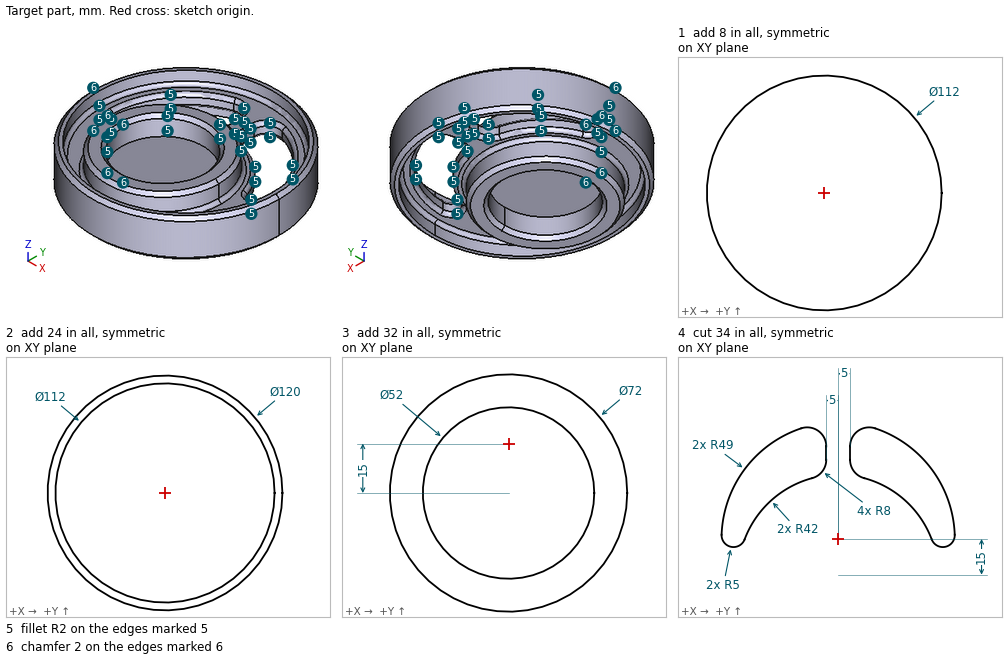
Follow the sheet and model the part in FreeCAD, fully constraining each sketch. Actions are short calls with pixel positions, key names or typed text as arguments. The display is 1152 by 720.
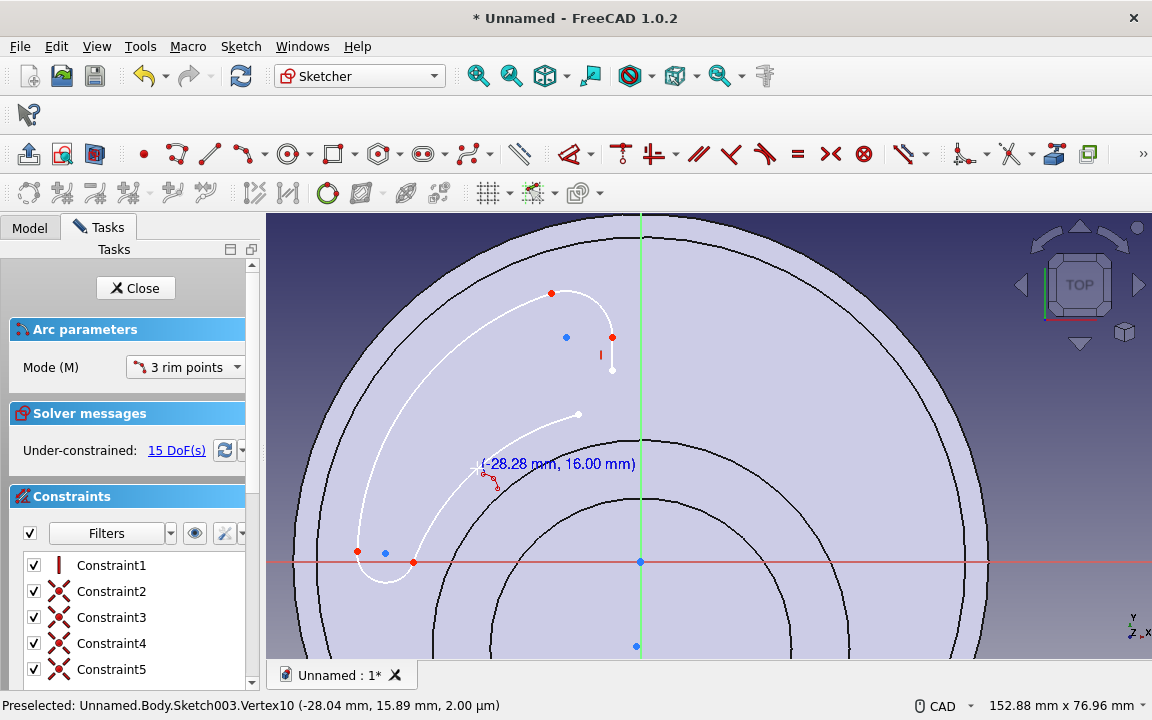
click(578, 415)
click(612, 370)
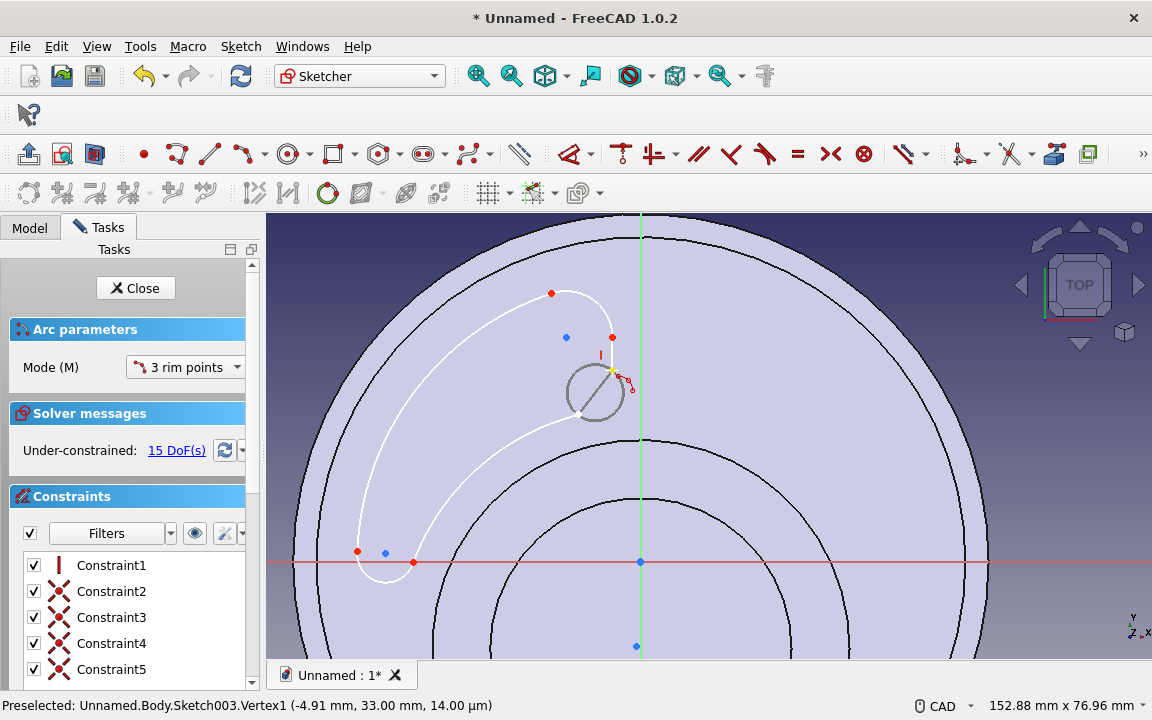
scroll(602, 397, up, 3)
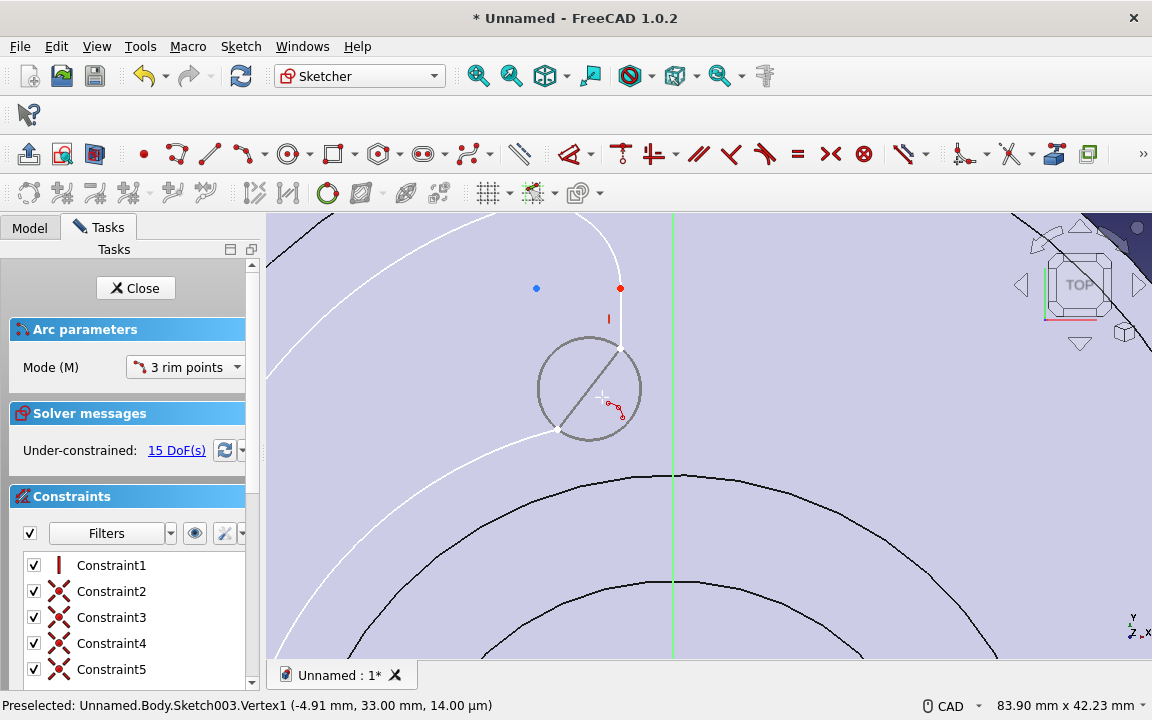
click(602, 397)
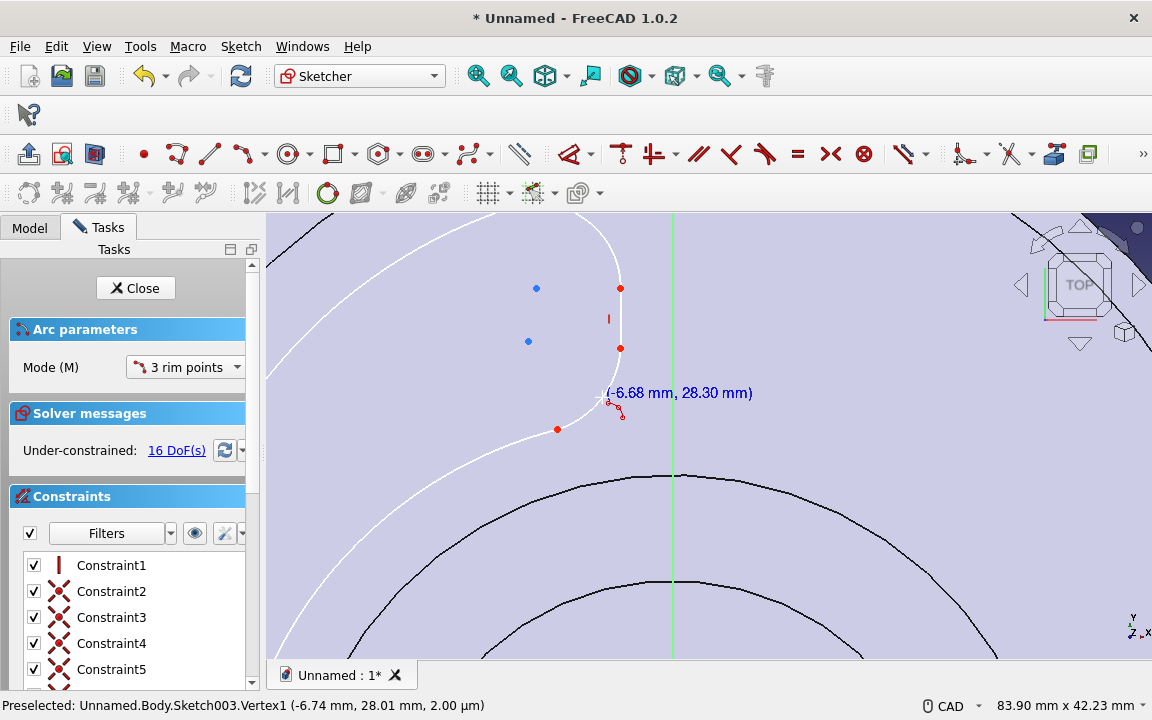
key(g)
key(l)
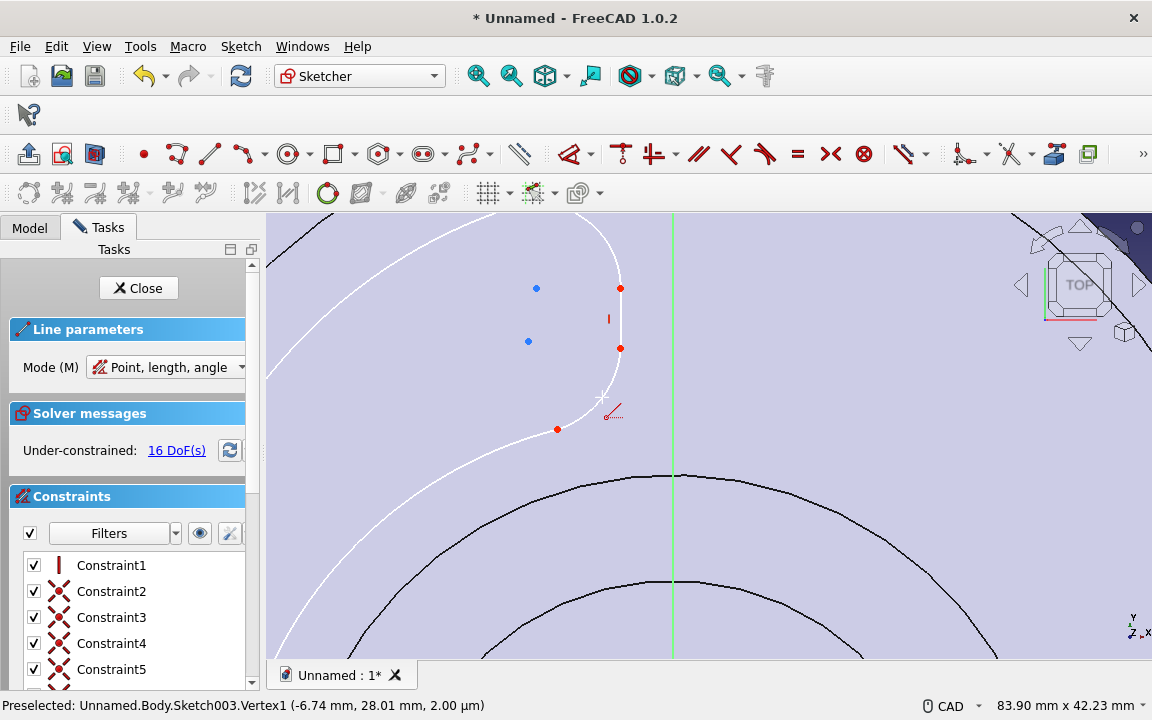
click(725, 286)
click(725, 345)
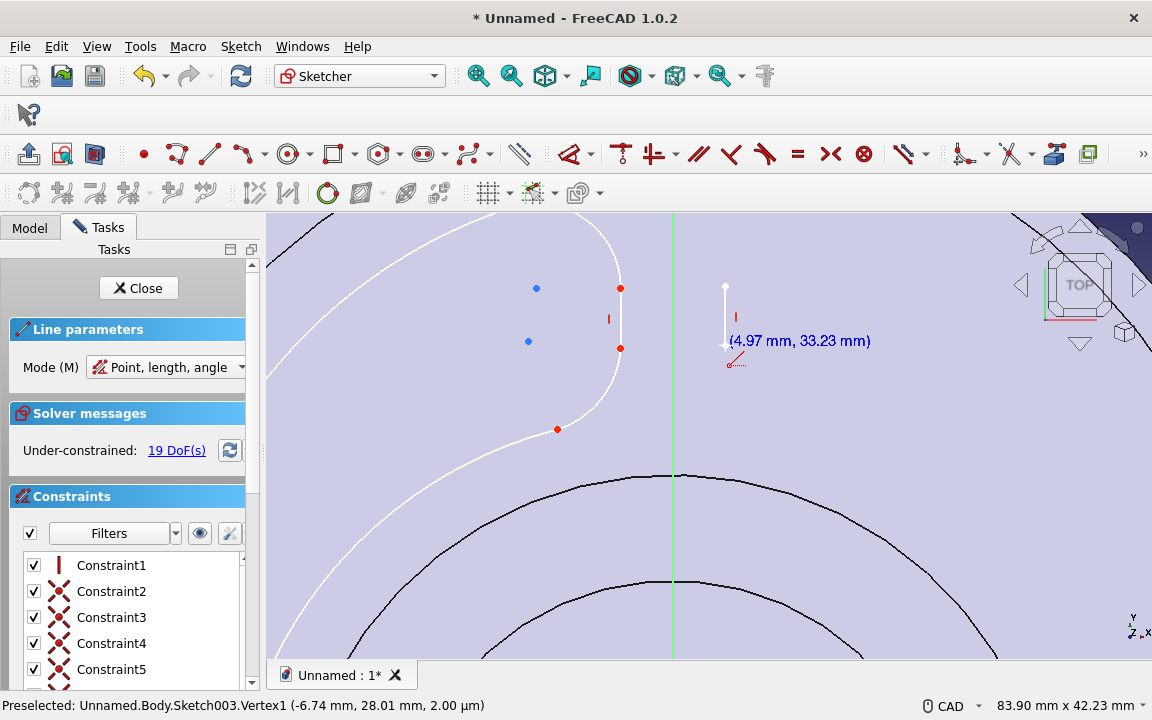
key(g)
key(3)
key(a)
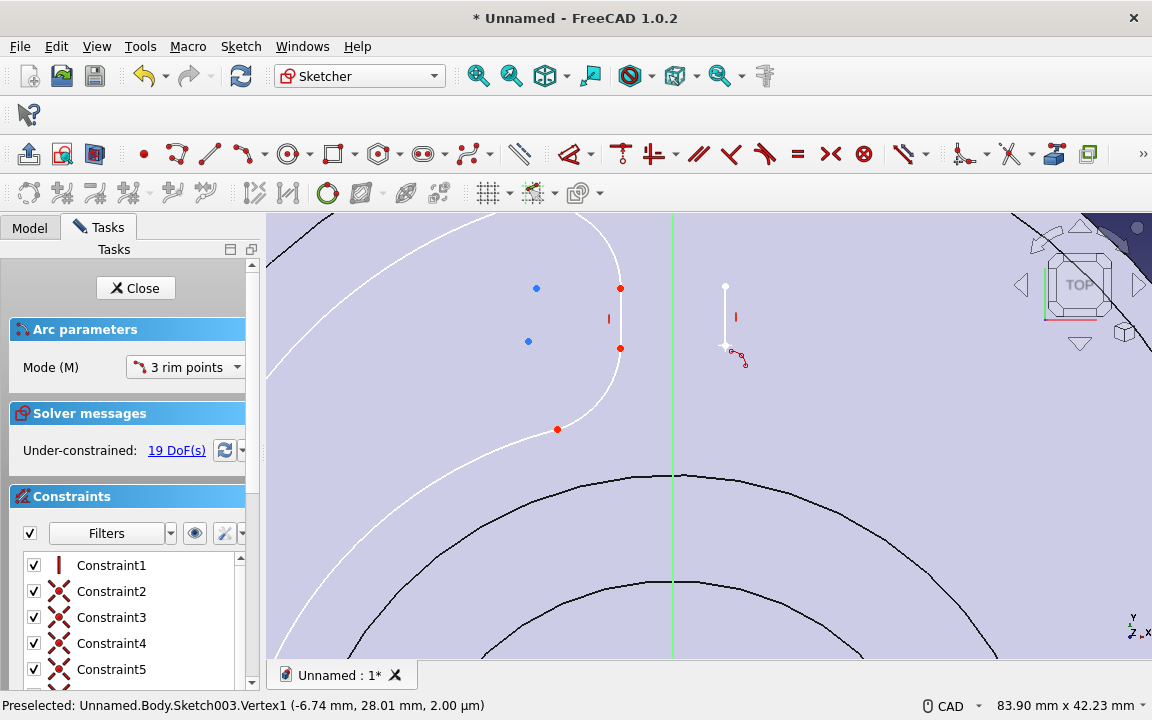
click(725, 346)
click(788, 427)
click(743, 397)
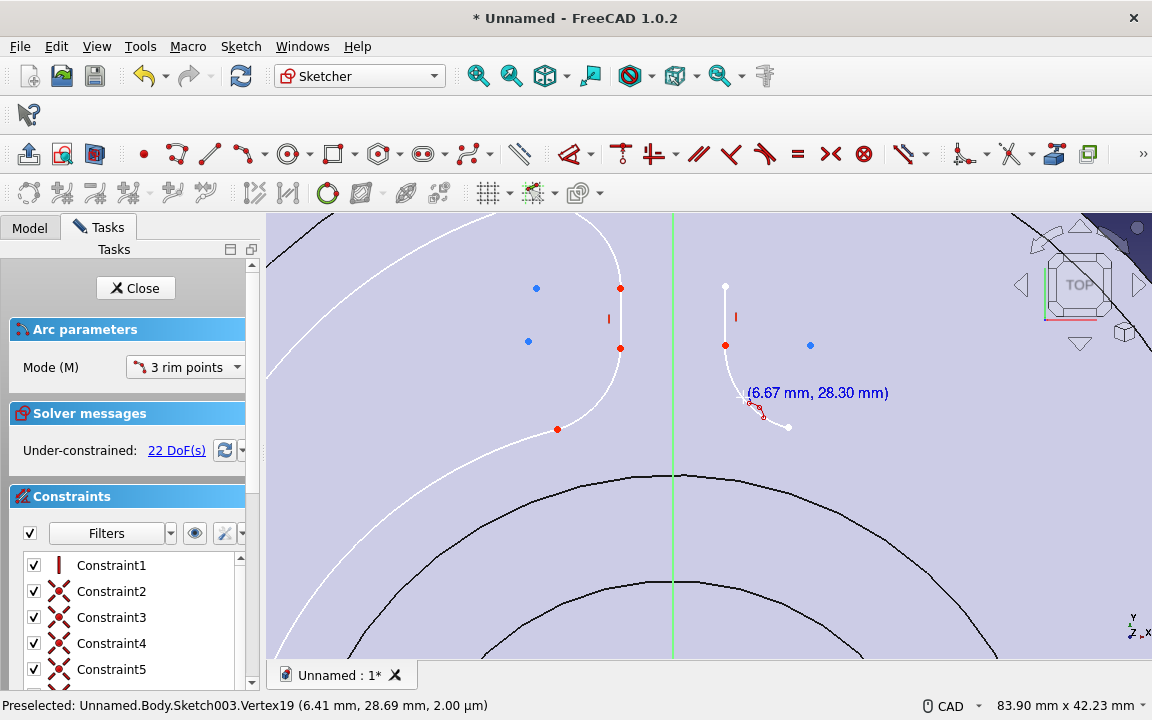
click(788, 428)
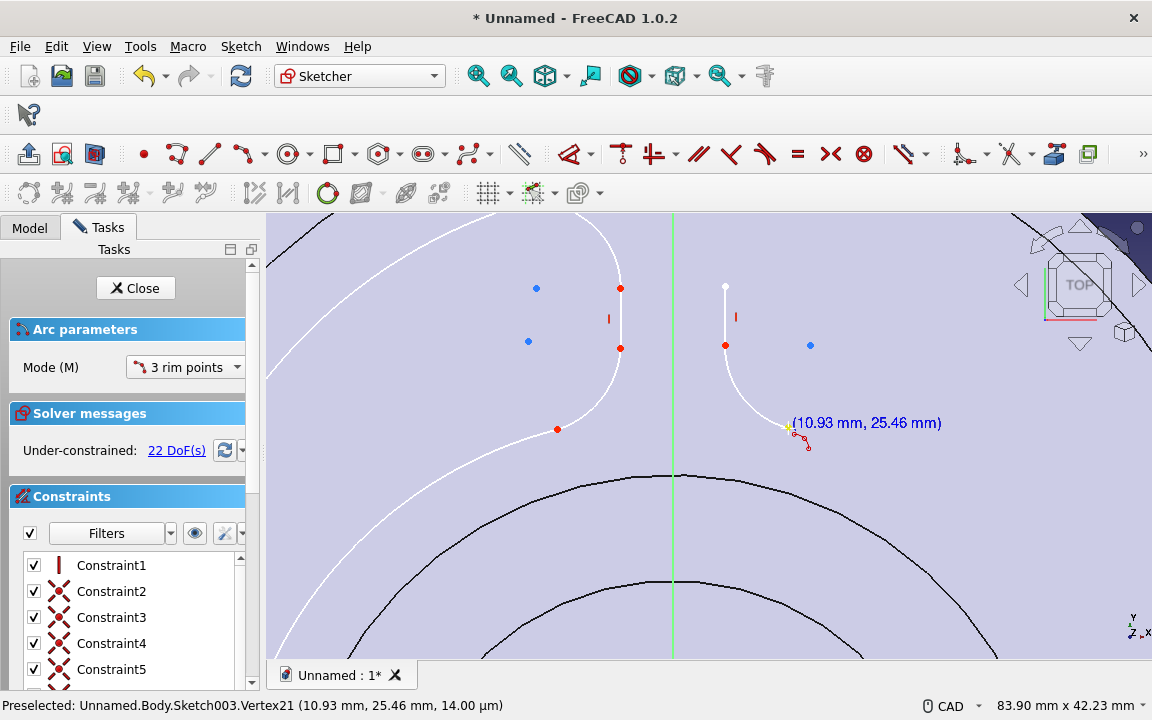
scroll(614, 409, down, 4)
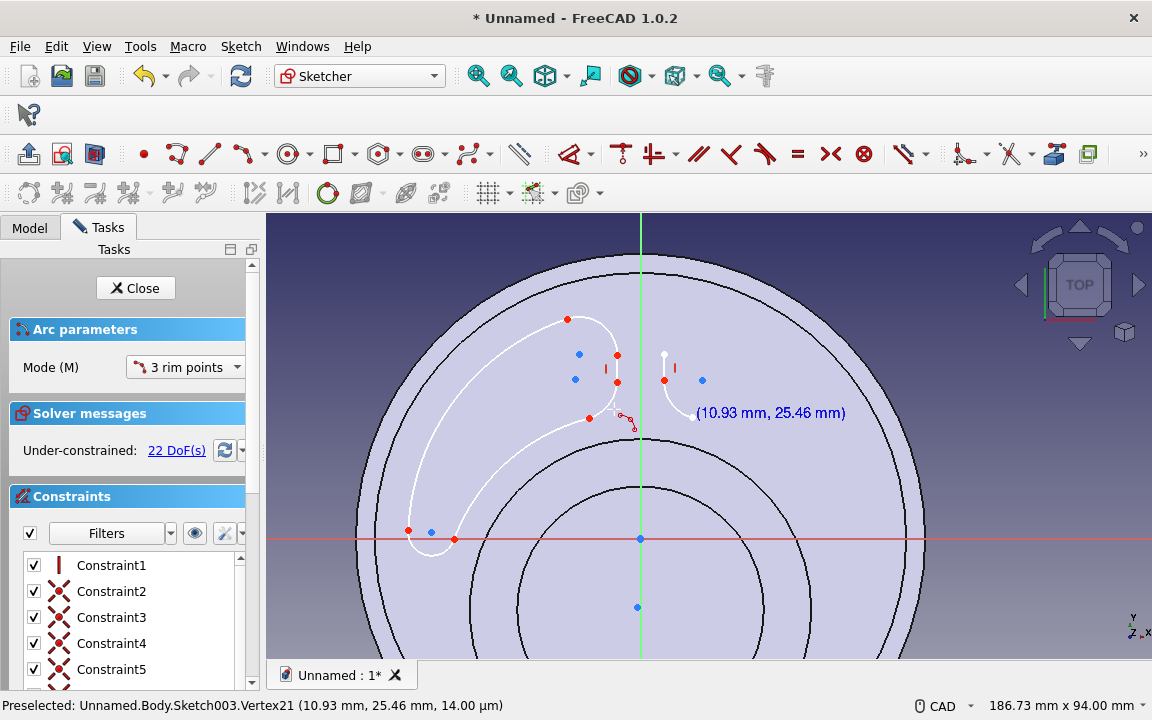
scroll(827, 539, up, 16)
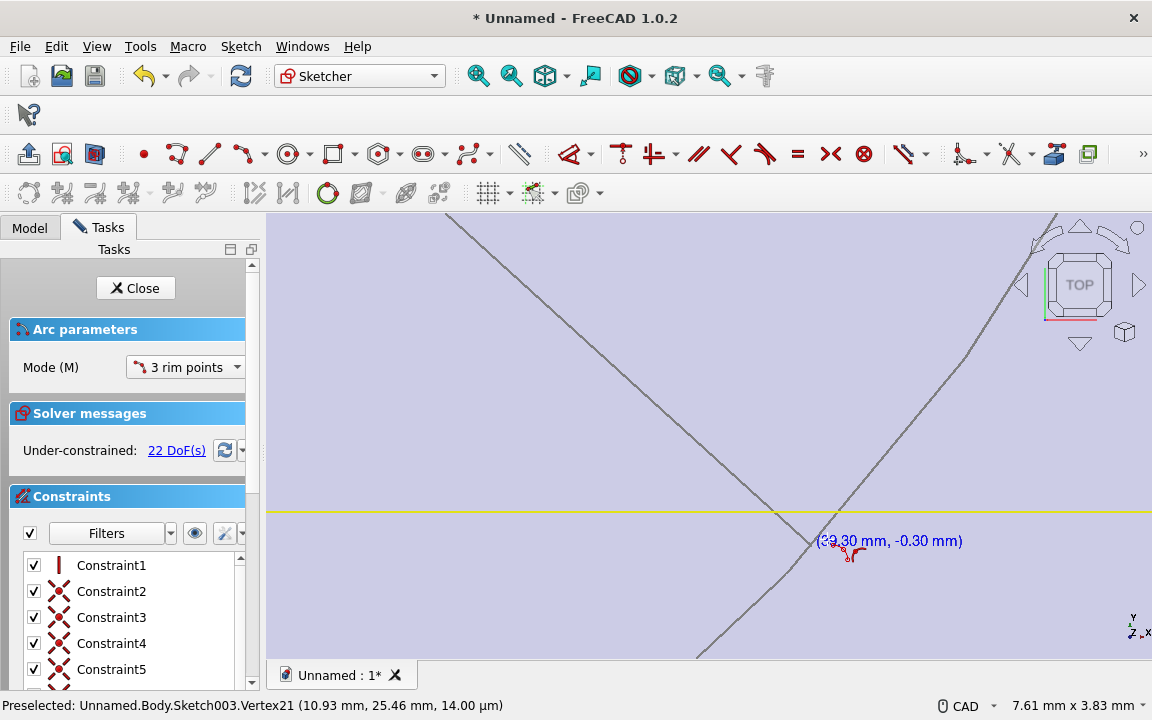
click(811, 531)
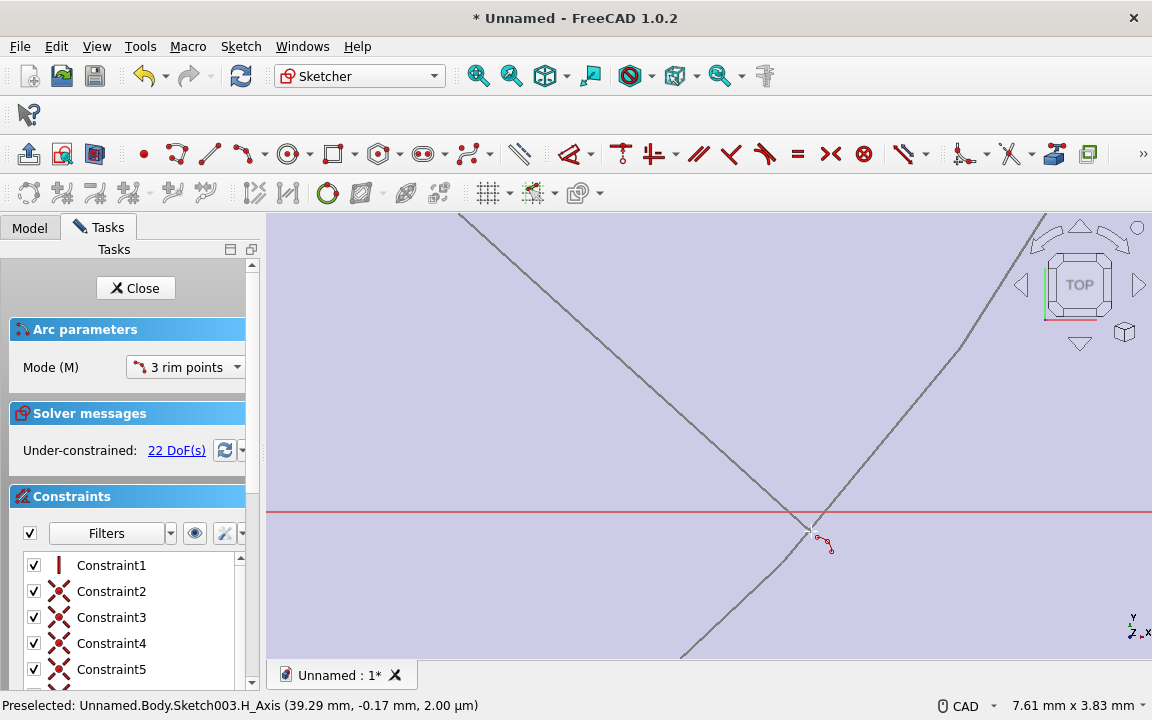
scroll(871, 564, down, 15)